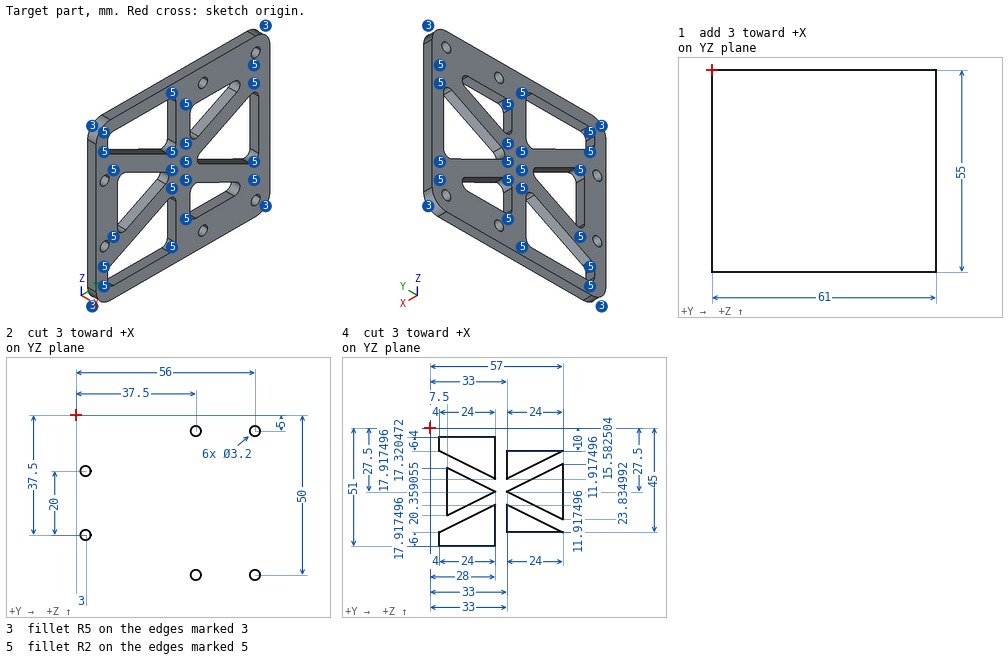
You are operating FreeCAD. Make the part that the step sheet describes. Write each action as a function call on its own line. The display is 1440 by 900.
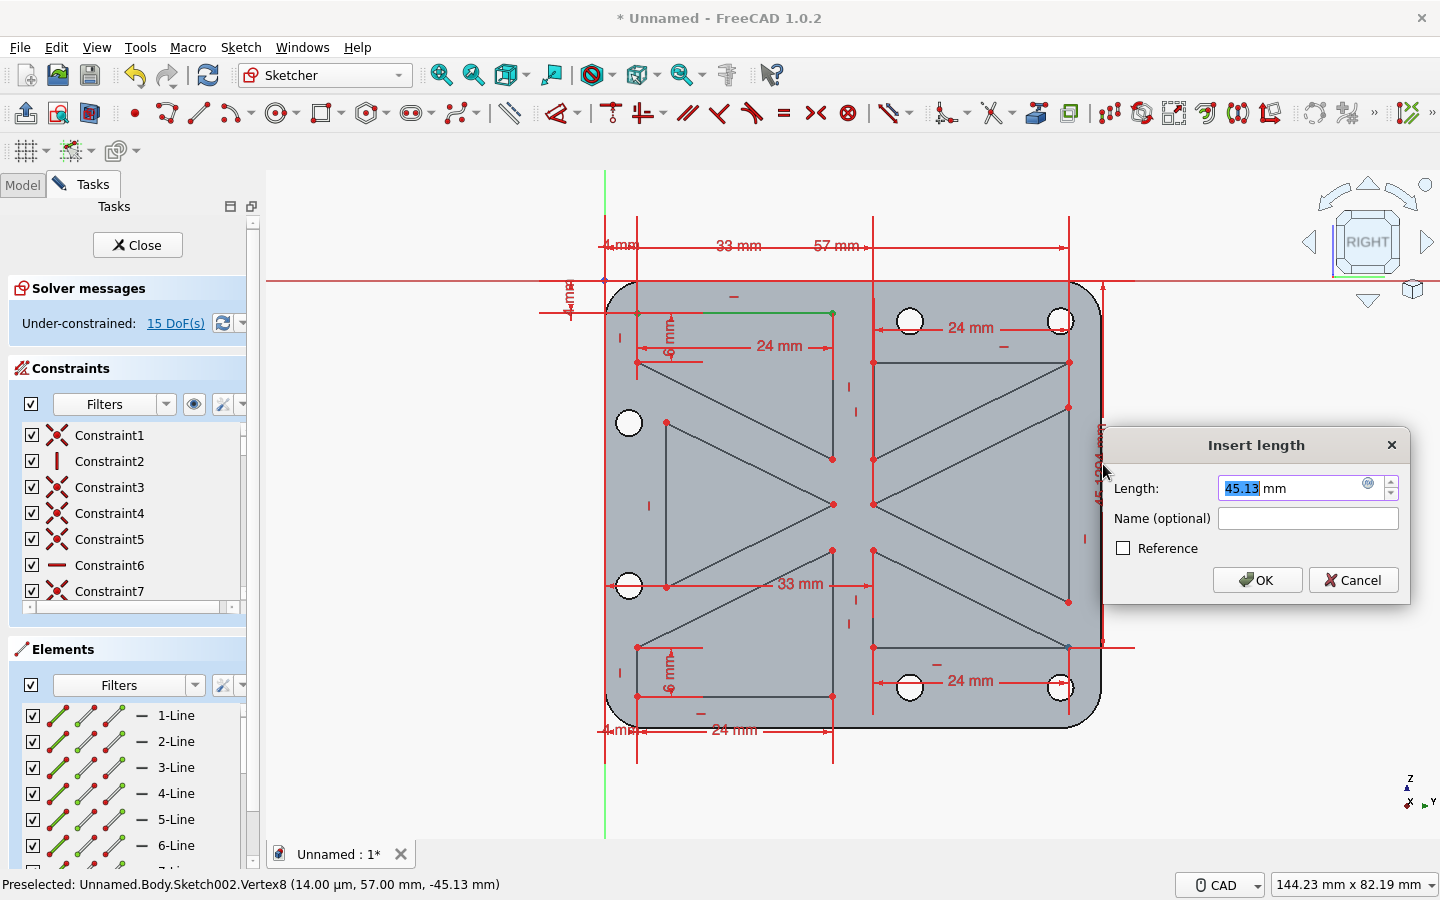
text(45)
key(Return)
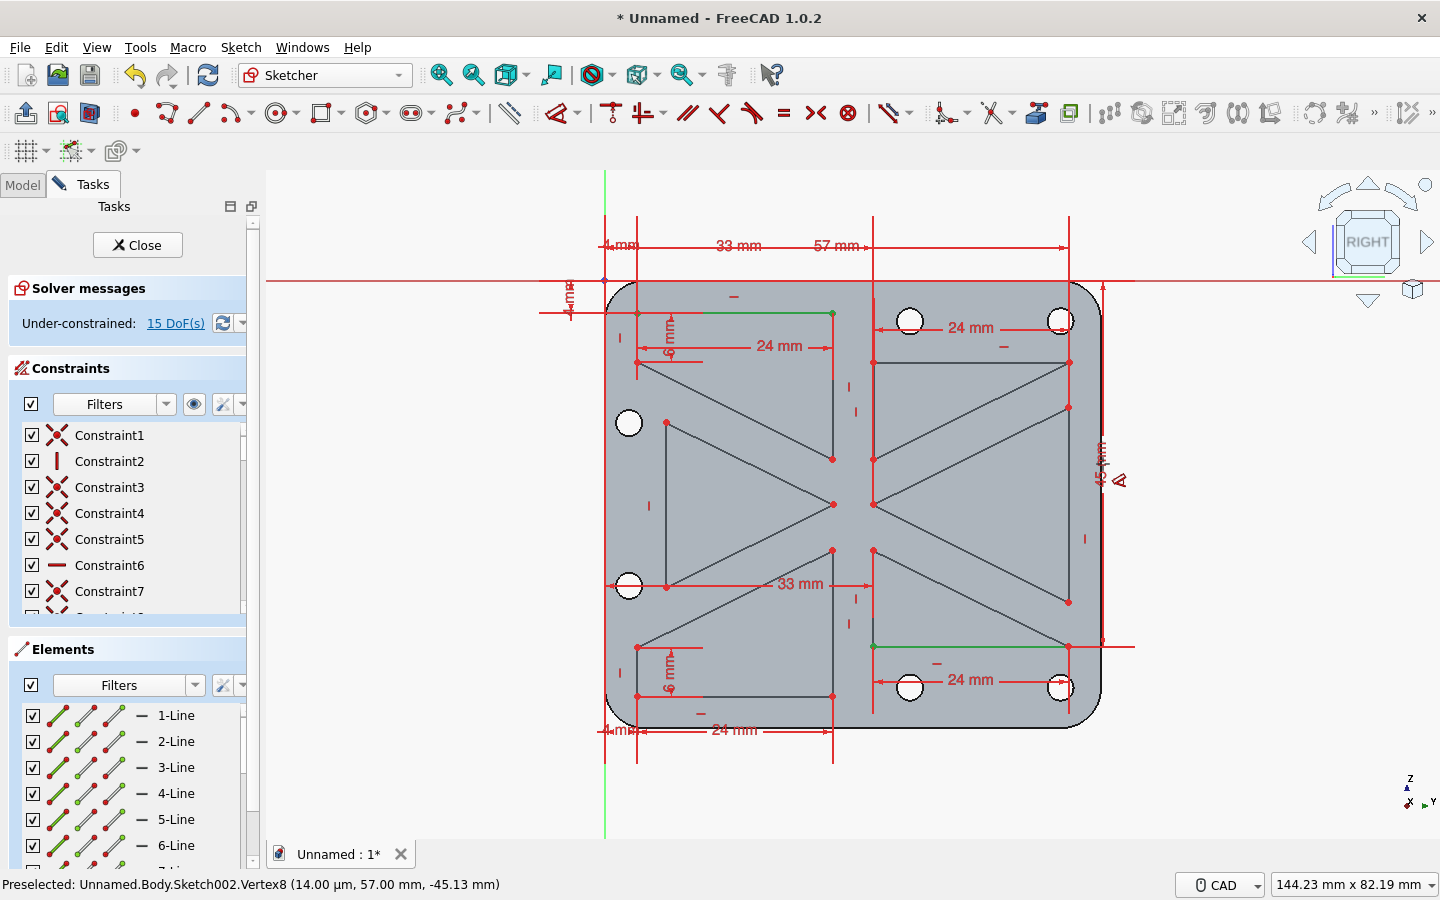
click(874, 363)
click(739, 397)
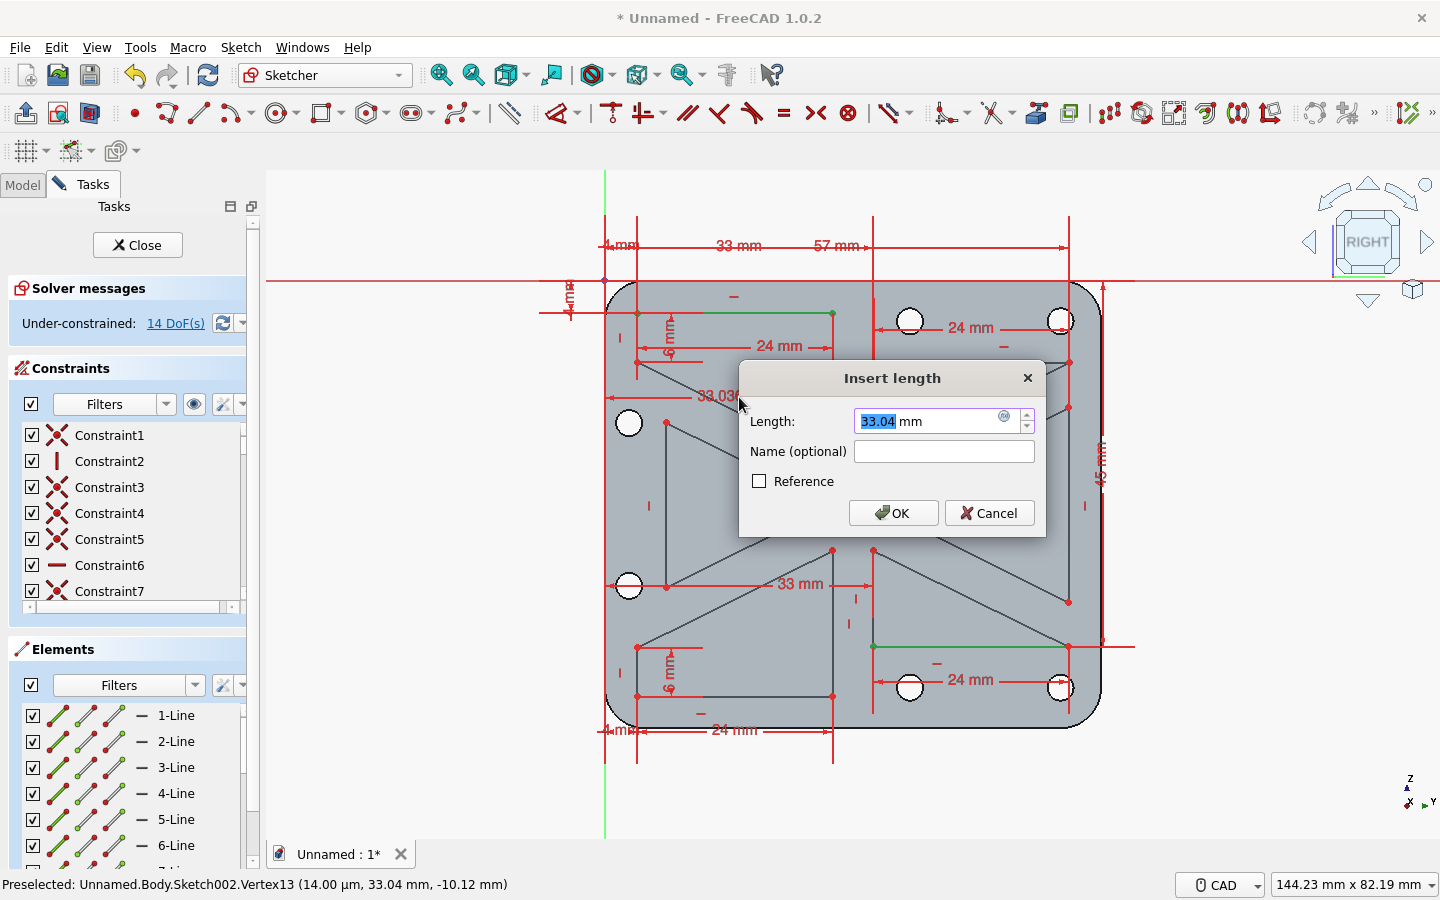
text(33)
key(Return)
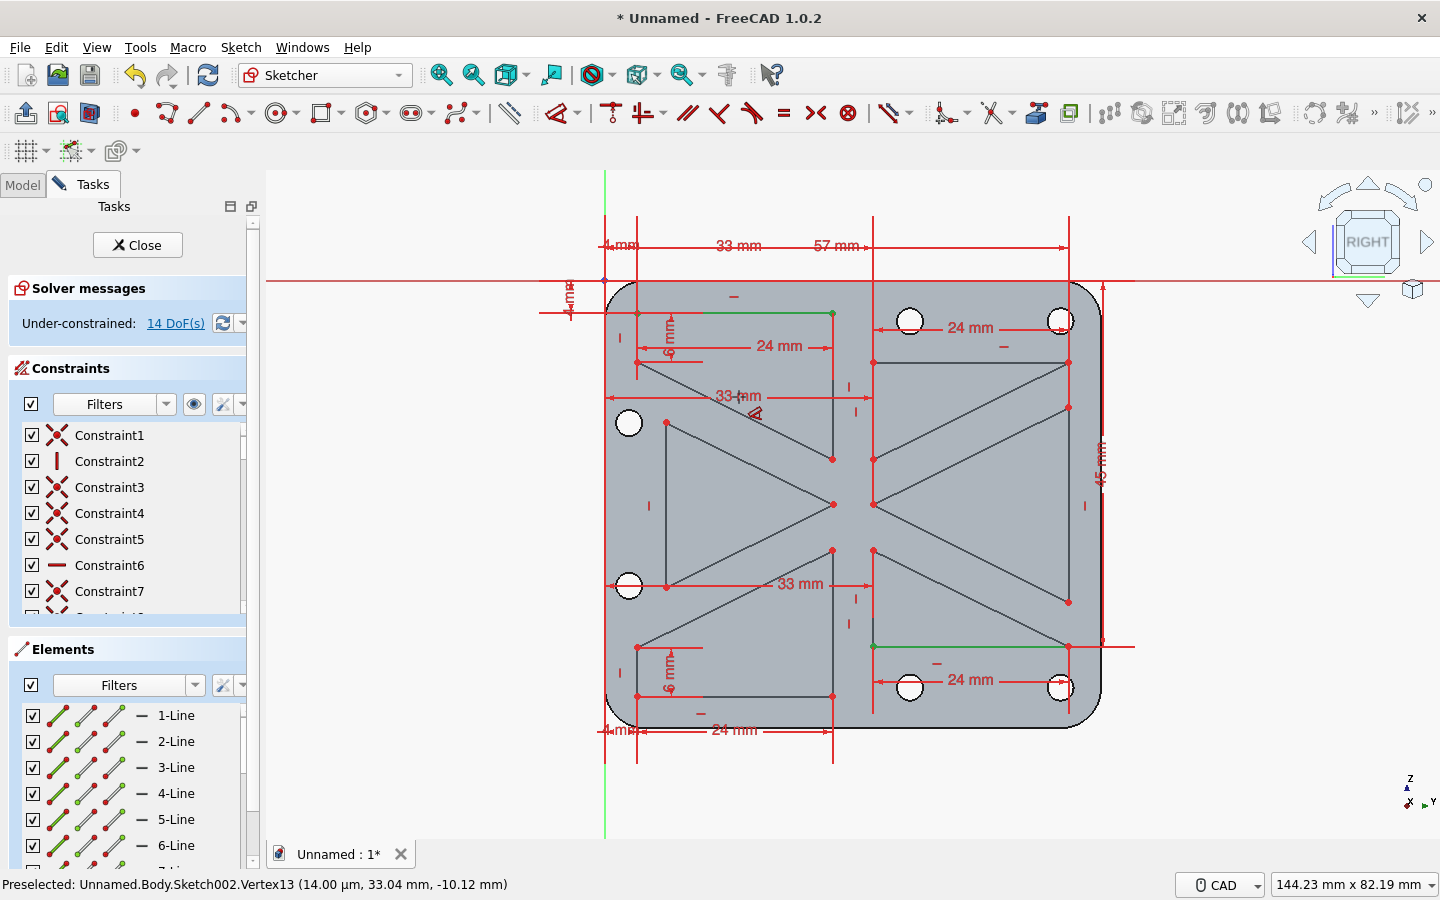
click(873, 363)
click(571, 322)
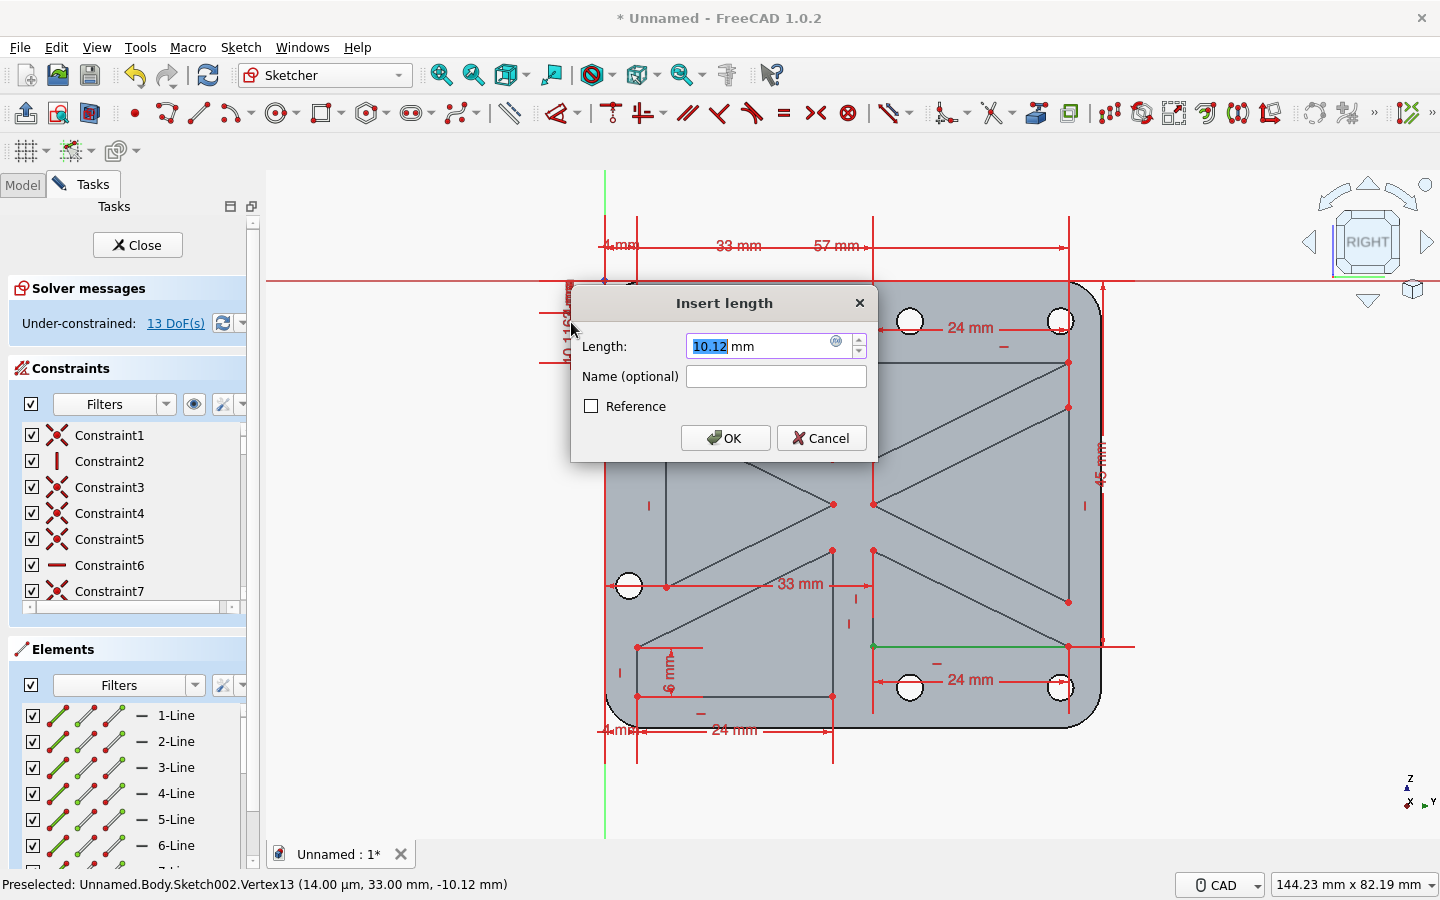
text(10)
key(Return)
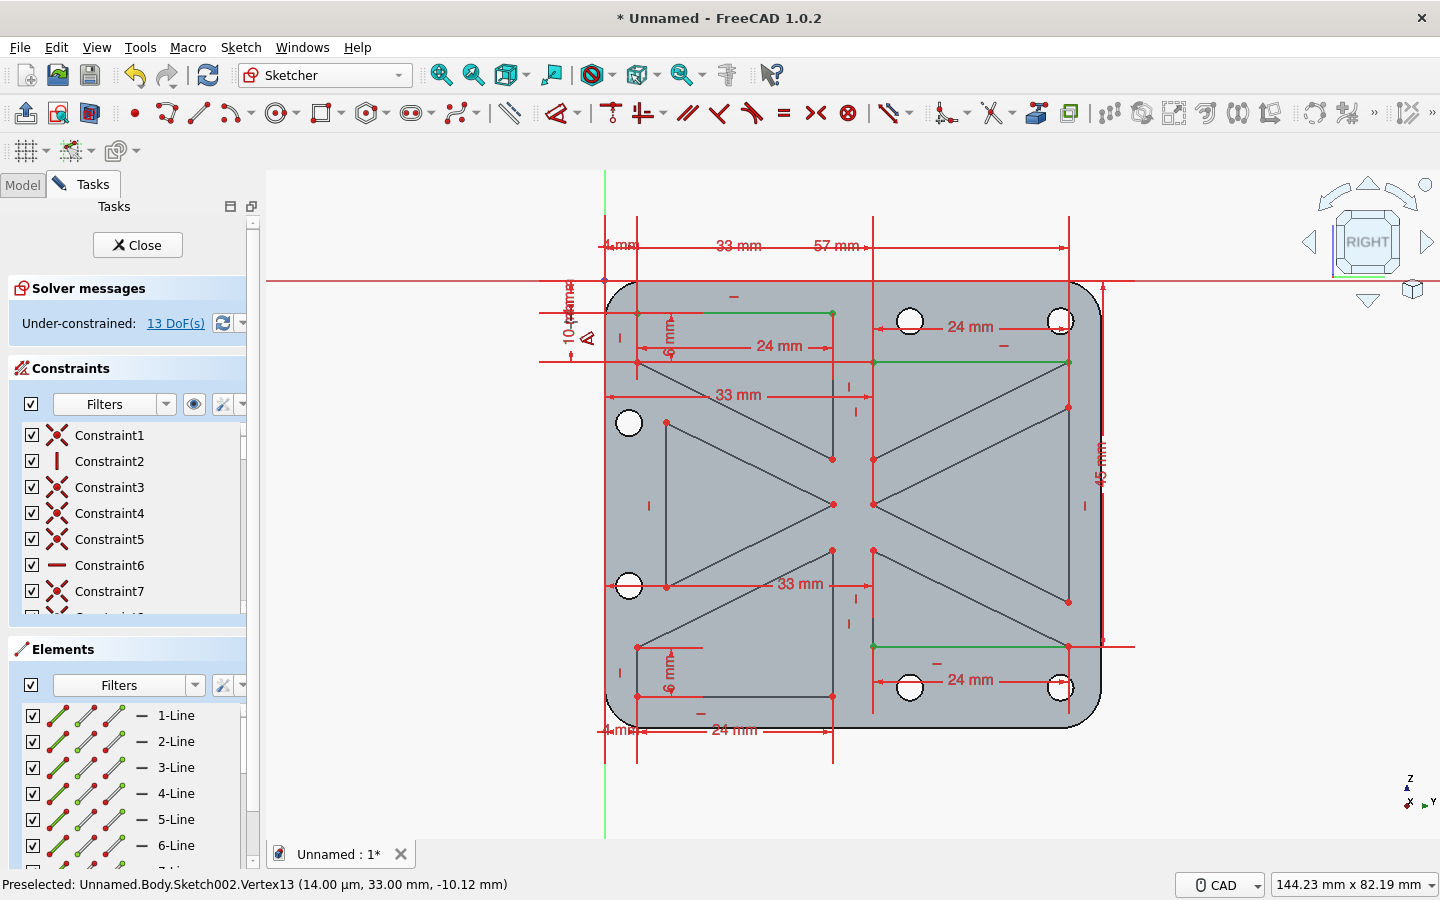
click(833, 505)
click(719, 539)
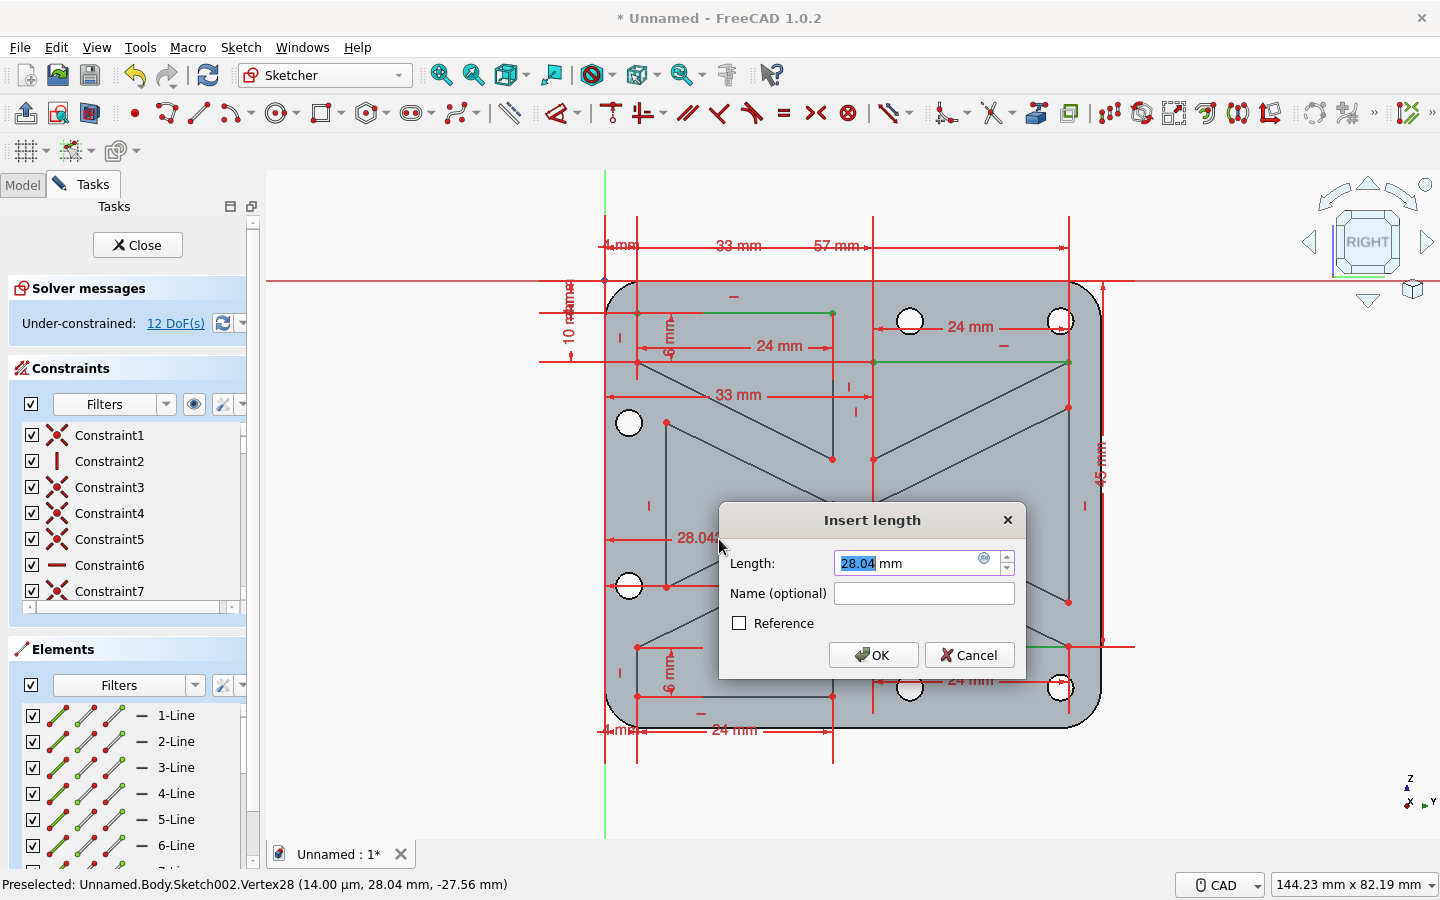
text(28)
key(Return)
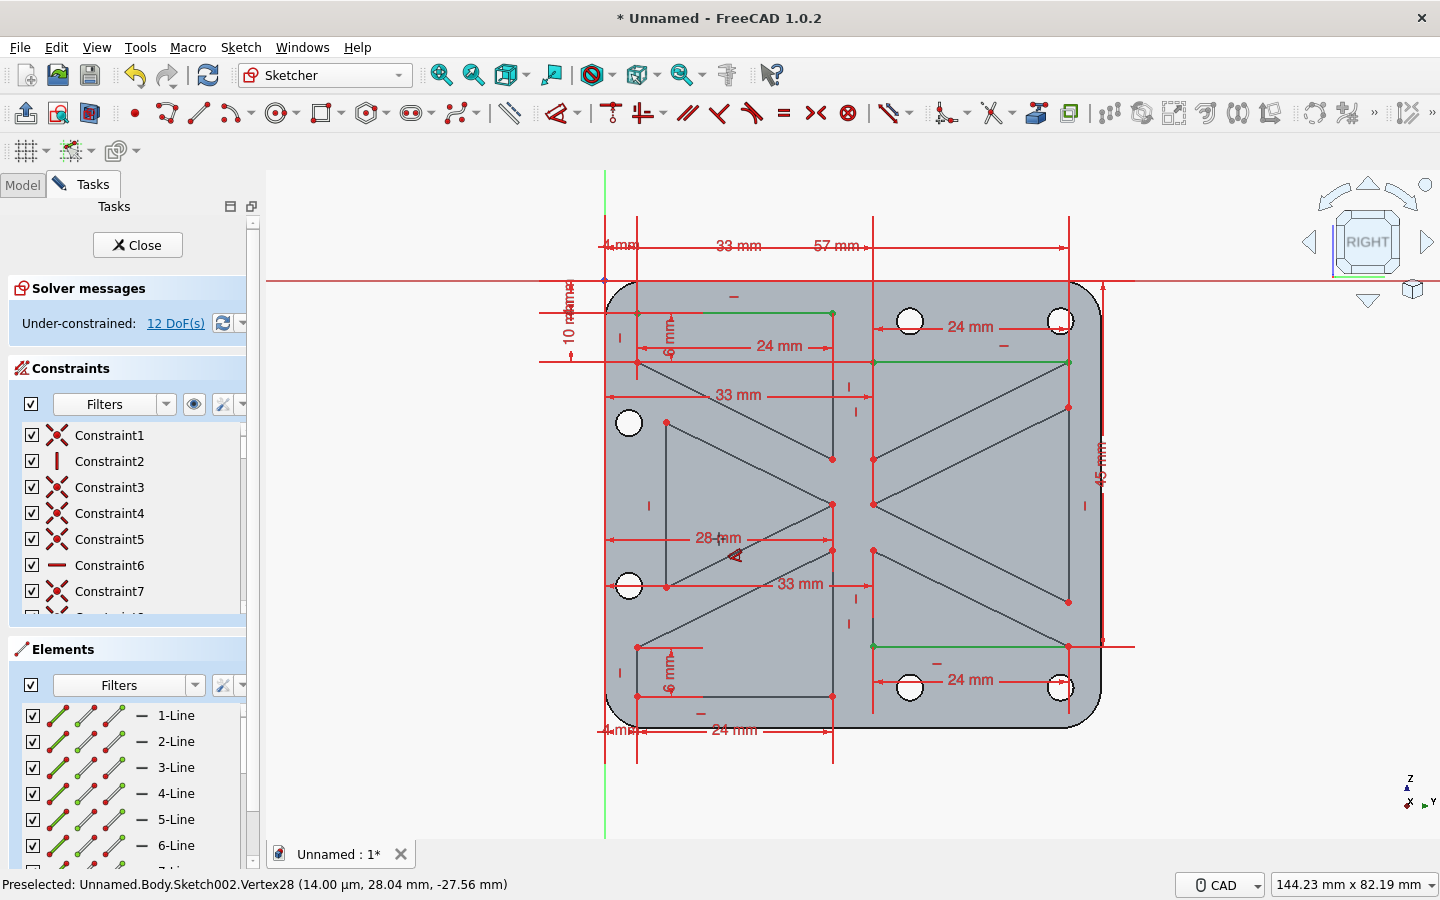
click(833, 697)
click(571, 489)